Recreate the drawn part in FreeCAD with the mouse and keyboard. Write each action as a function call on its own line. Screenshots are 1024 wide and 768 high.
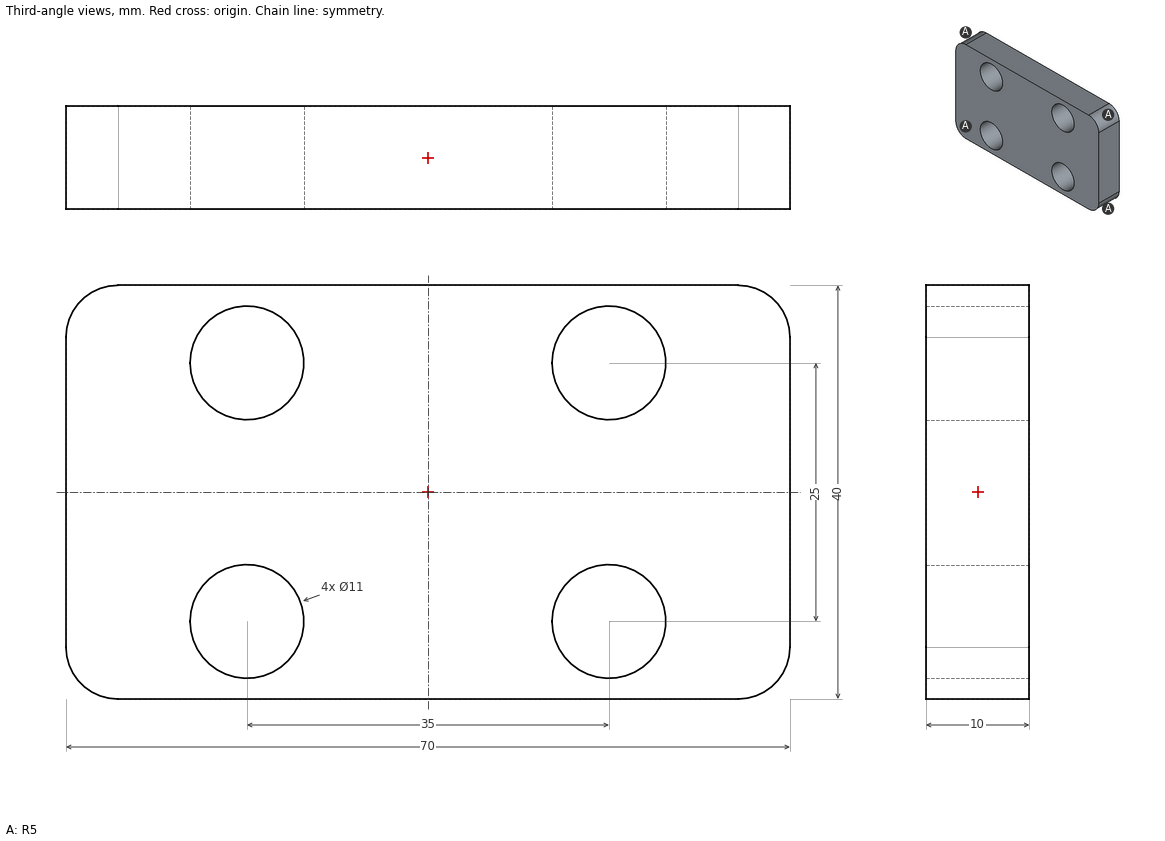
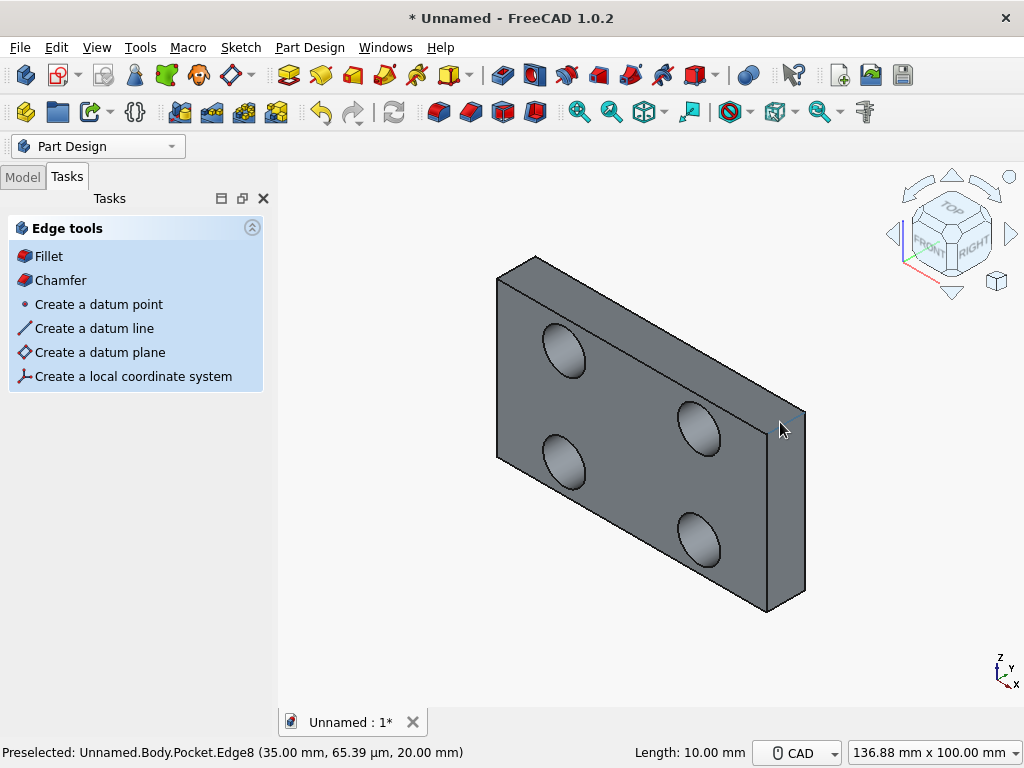
key(2)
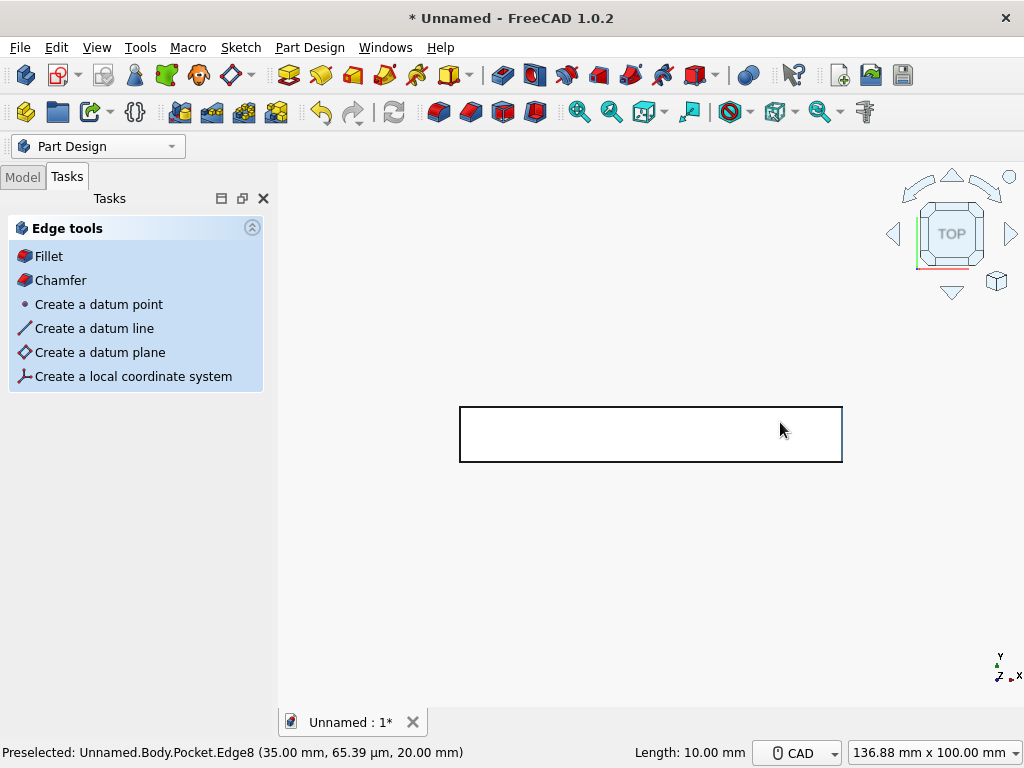
click(460, 433, ctrl)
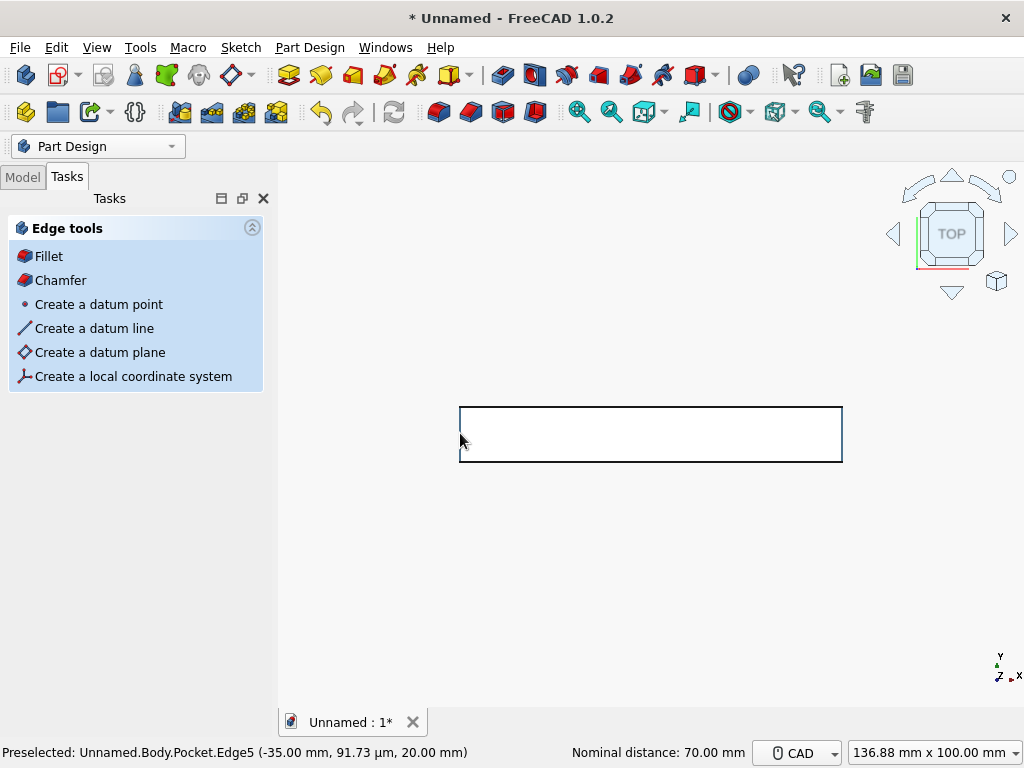
key(1)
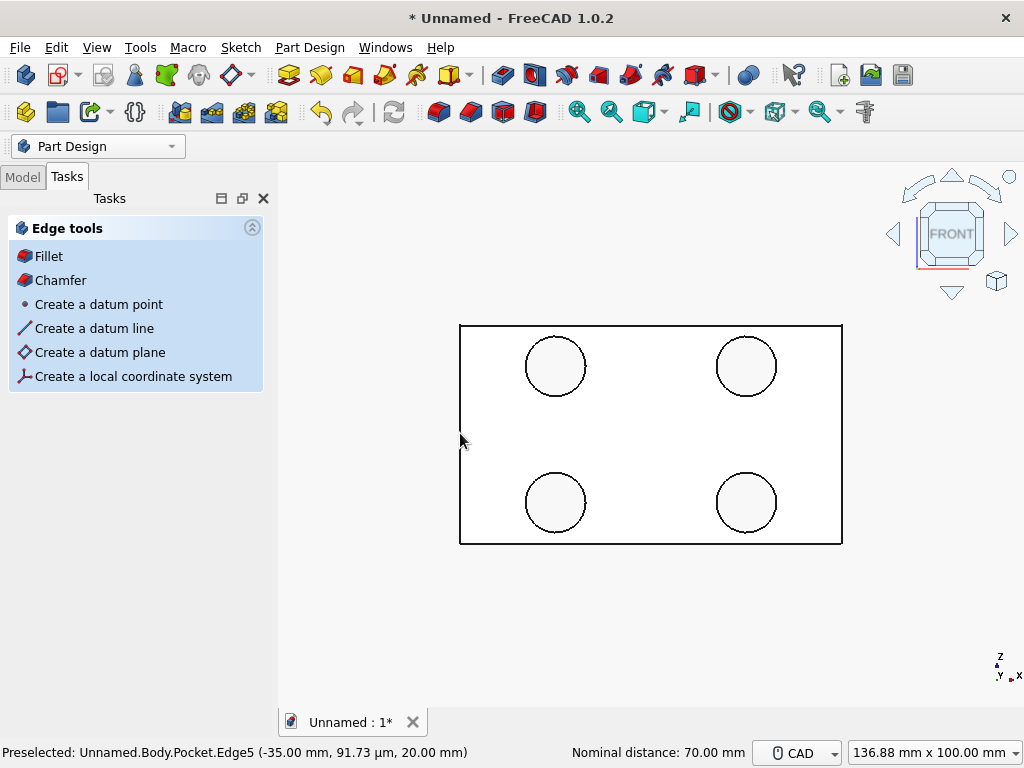
key(3)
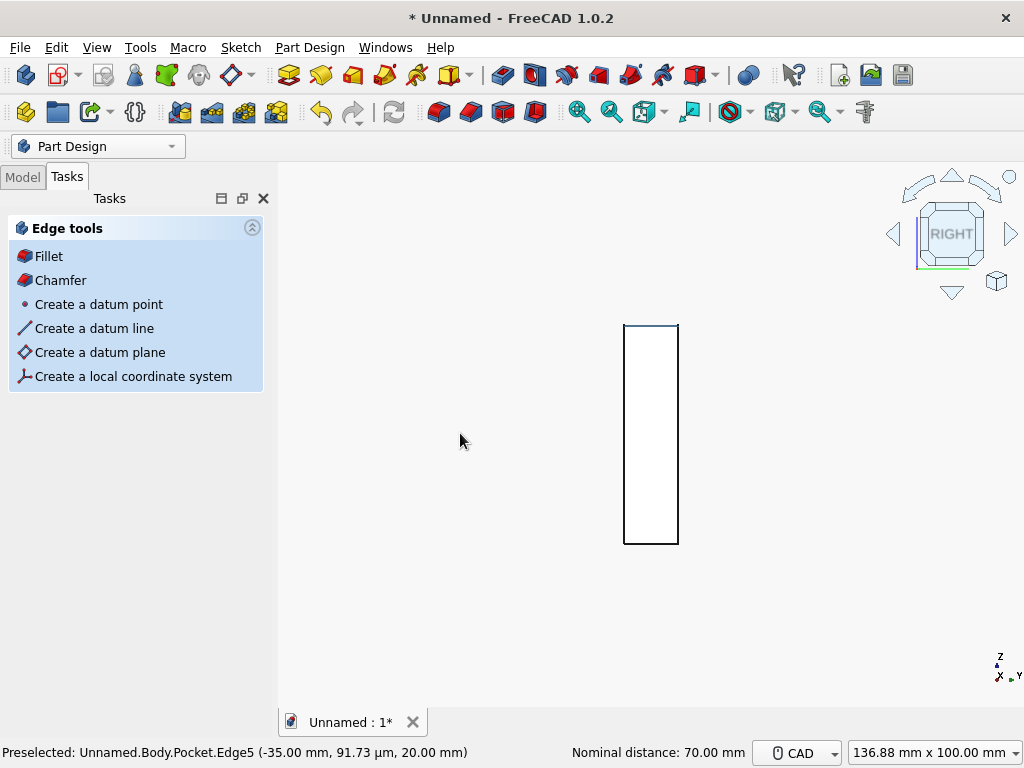
click(580, 112)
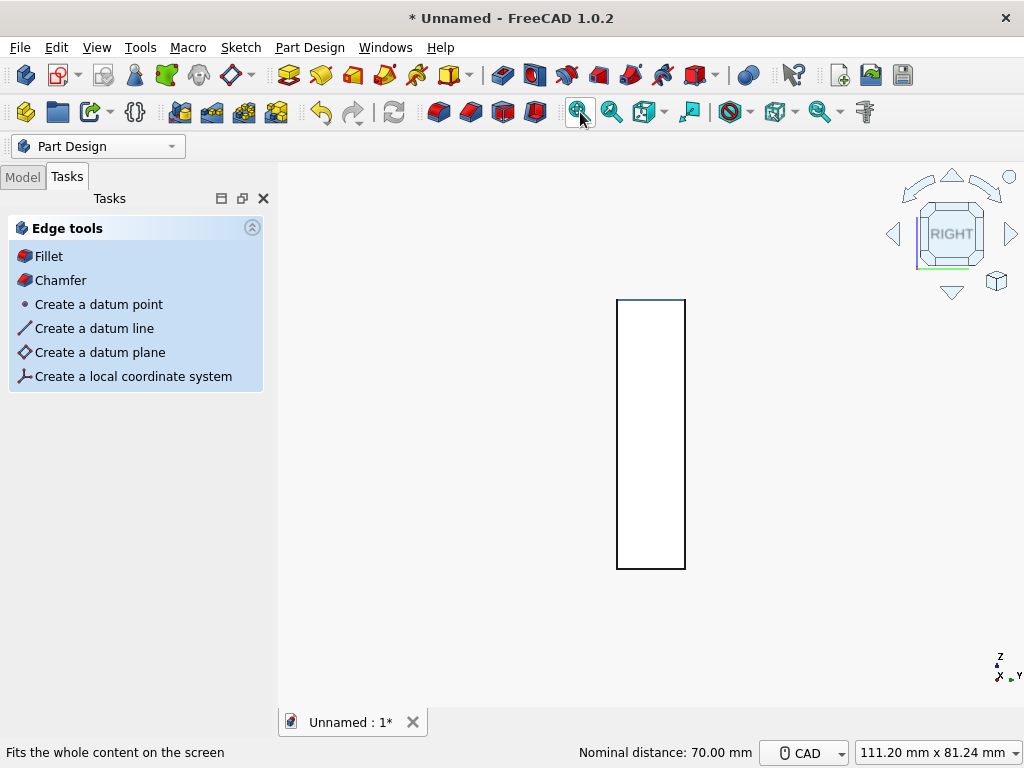
click(651, 568, ctrl)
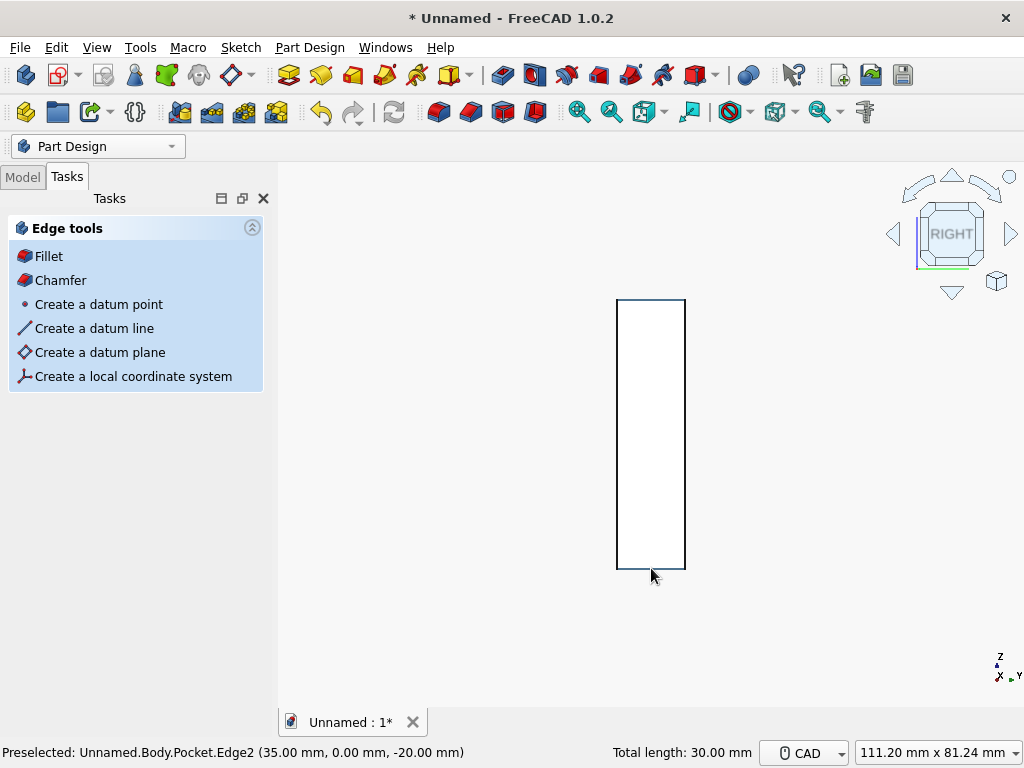
key(5)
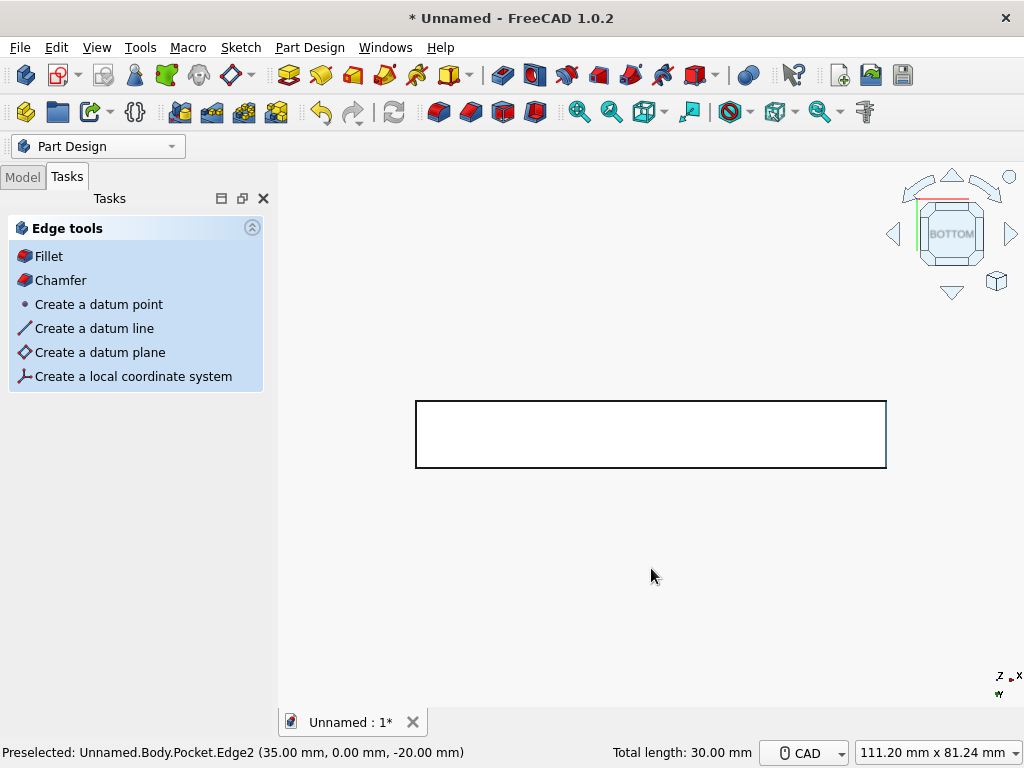
click(416, 433, ctrl)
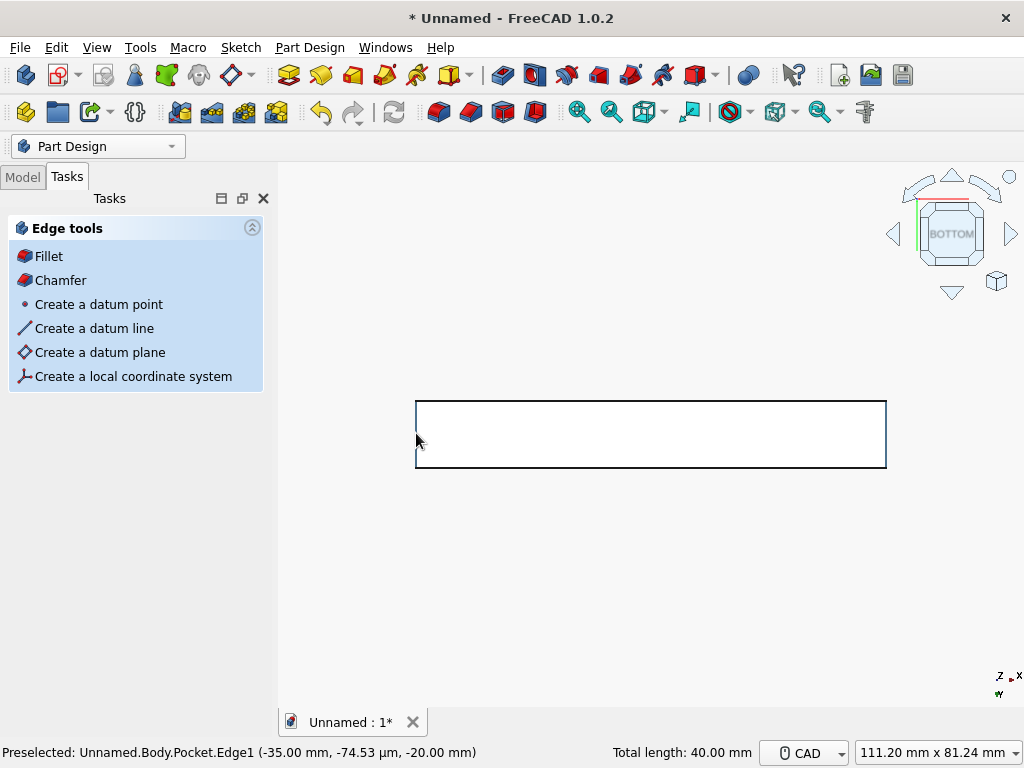
click(440, 112)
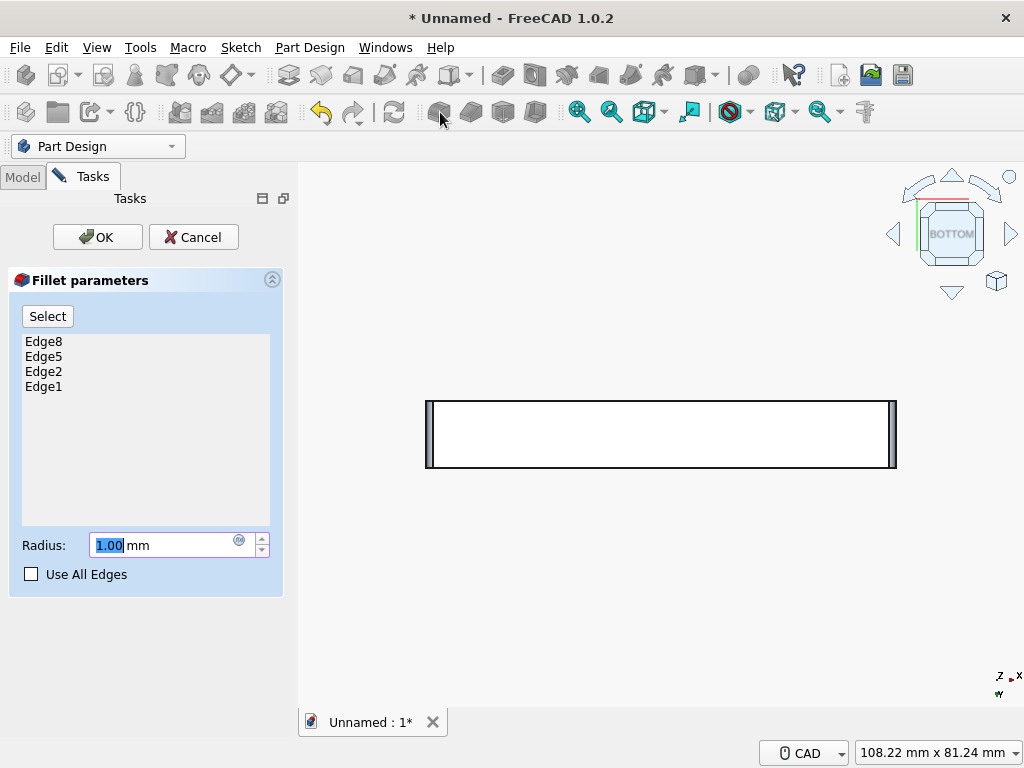
text(5)
key(Tab)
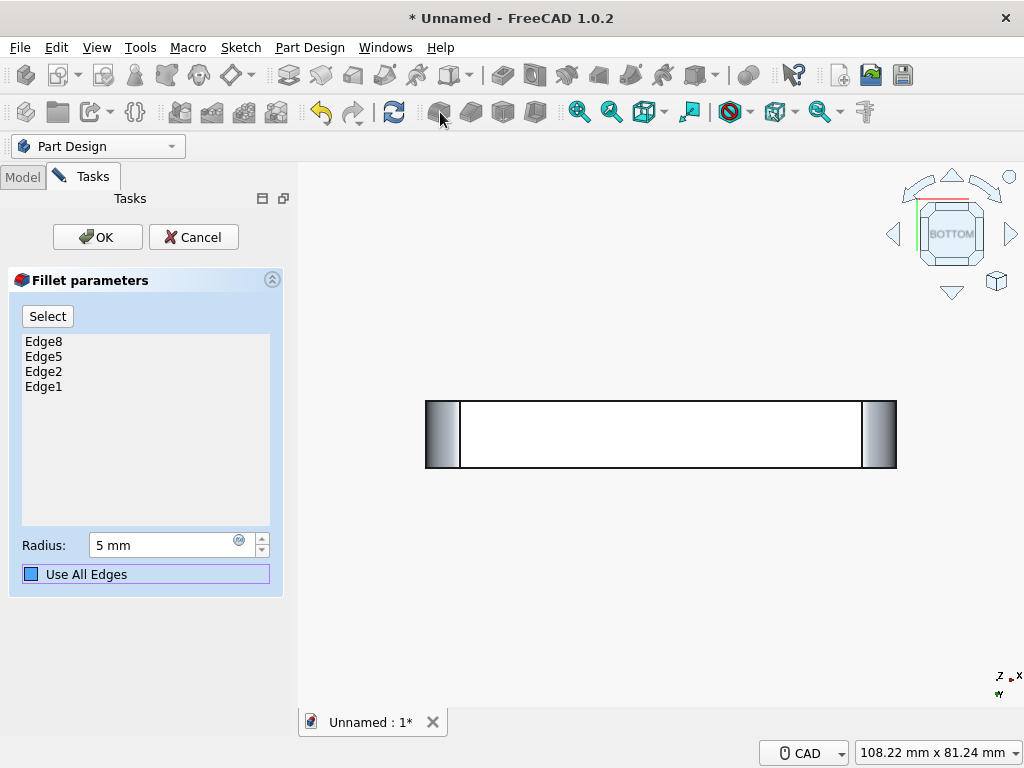
click(98, 237)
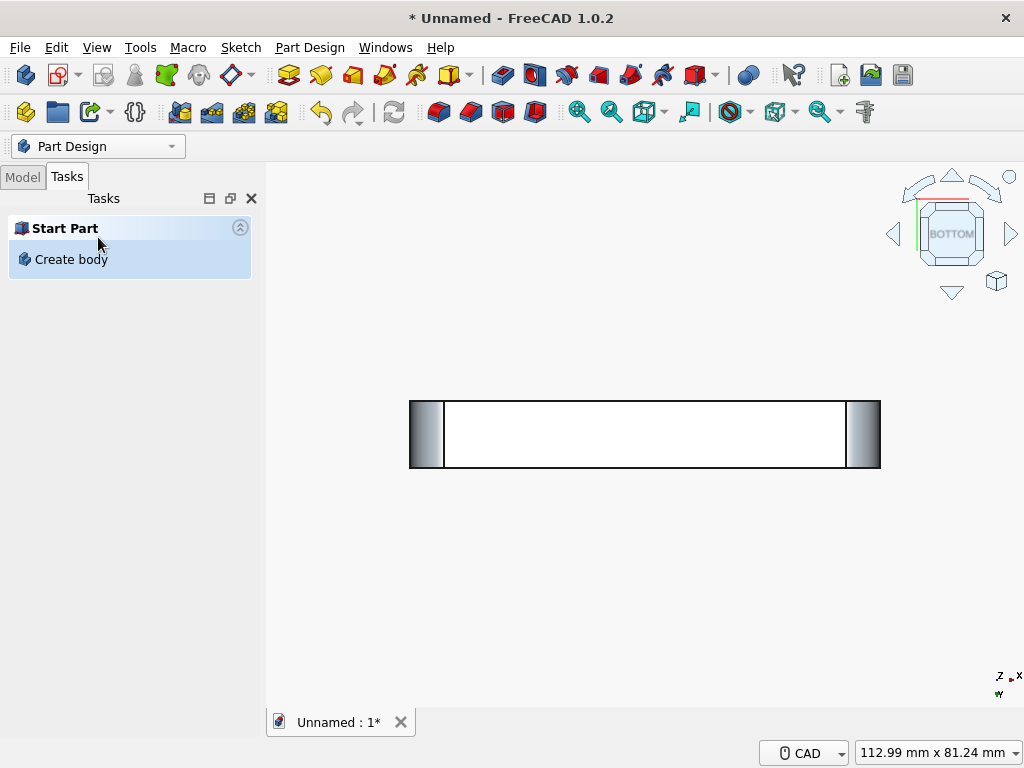
key(0)